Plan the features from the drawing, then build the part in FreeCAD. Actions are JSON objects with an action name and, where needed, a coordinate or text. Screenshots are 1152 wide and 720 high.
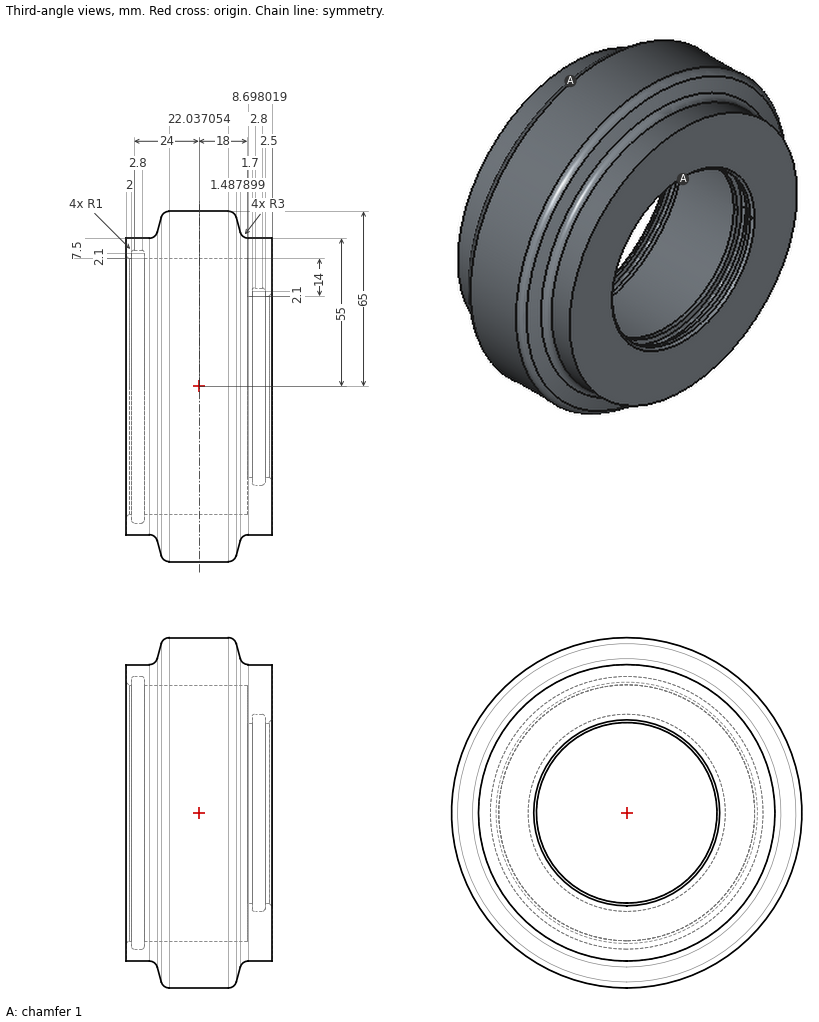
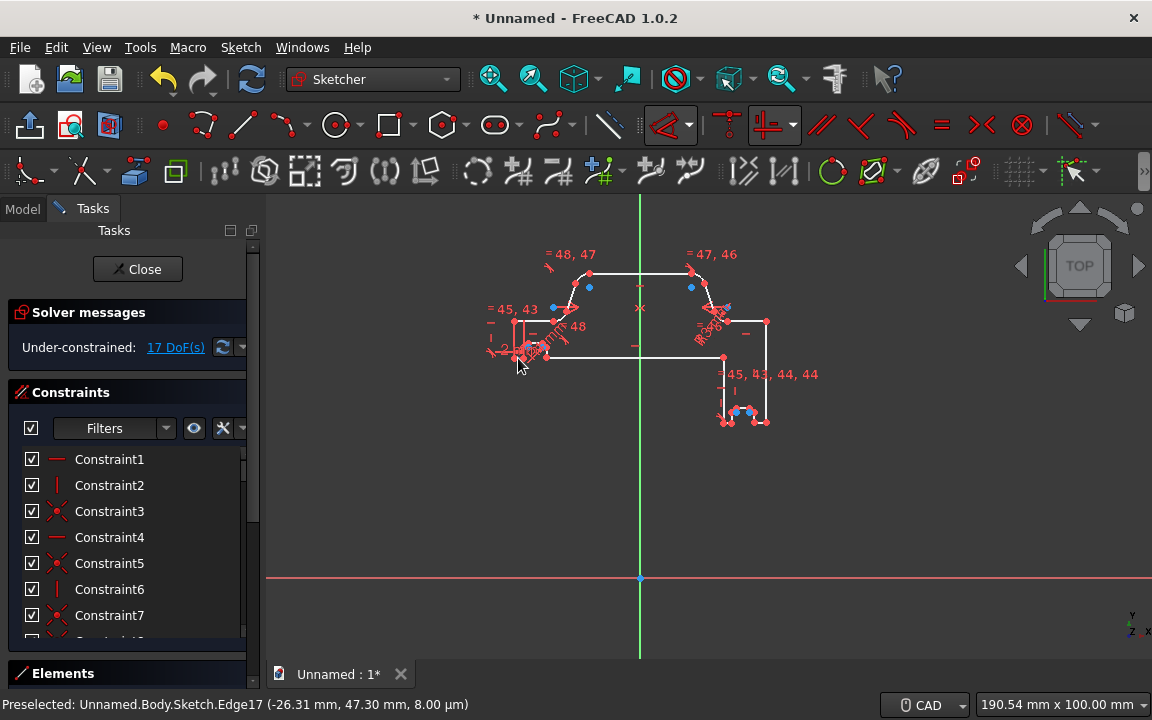
{"action": "scroll", "coordinate": [724, 377], "scroll_direction": "up", "scroll_amount": 4}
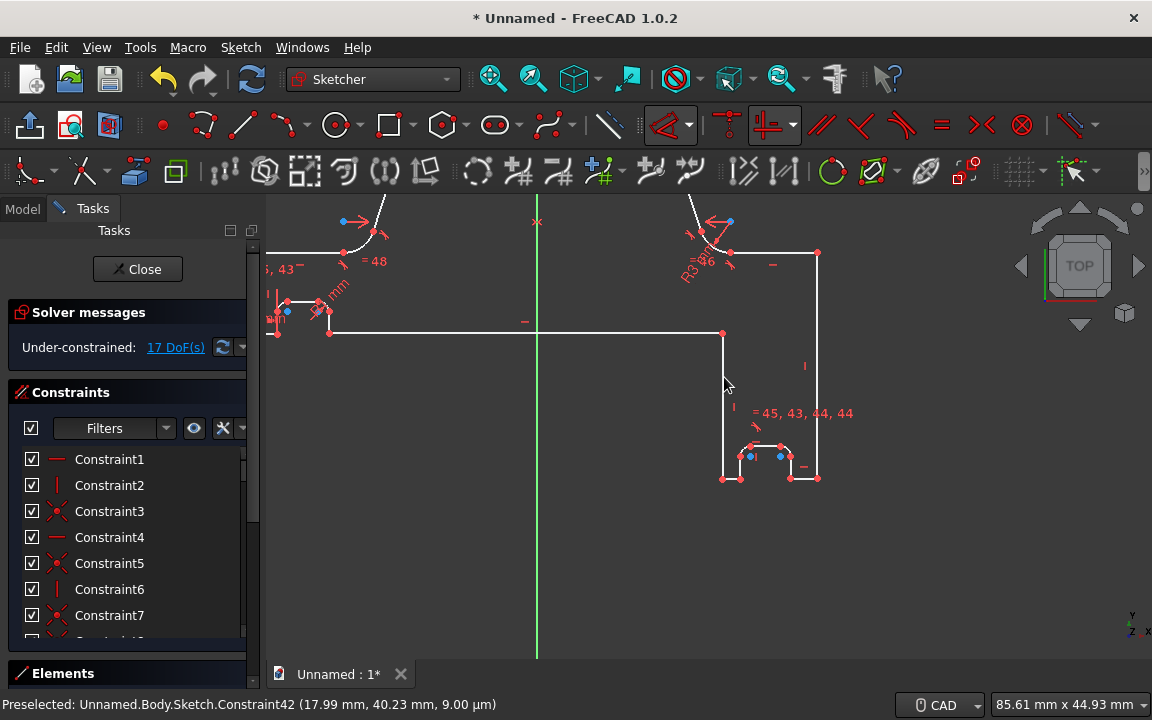
{"action": "left_click", "coordinate": [723, 377]}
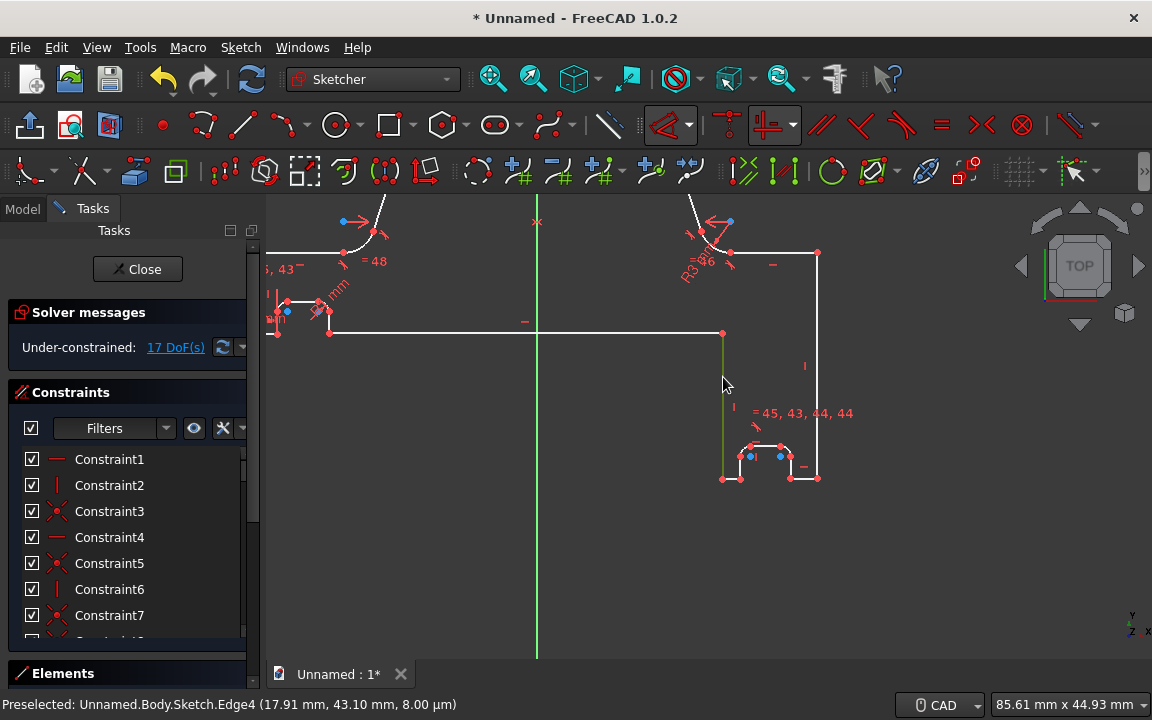
{"action": "key", "text": "i"}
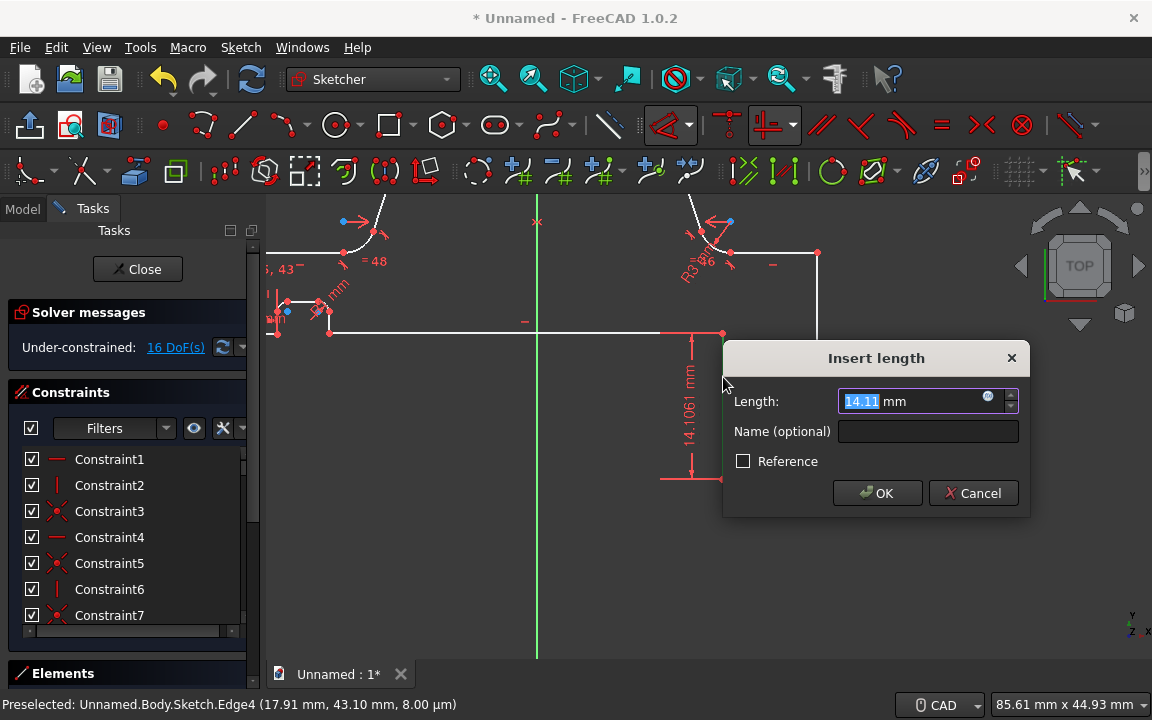
{"action": "type", "text": "14"}
{"action": "key", "text": "Return"}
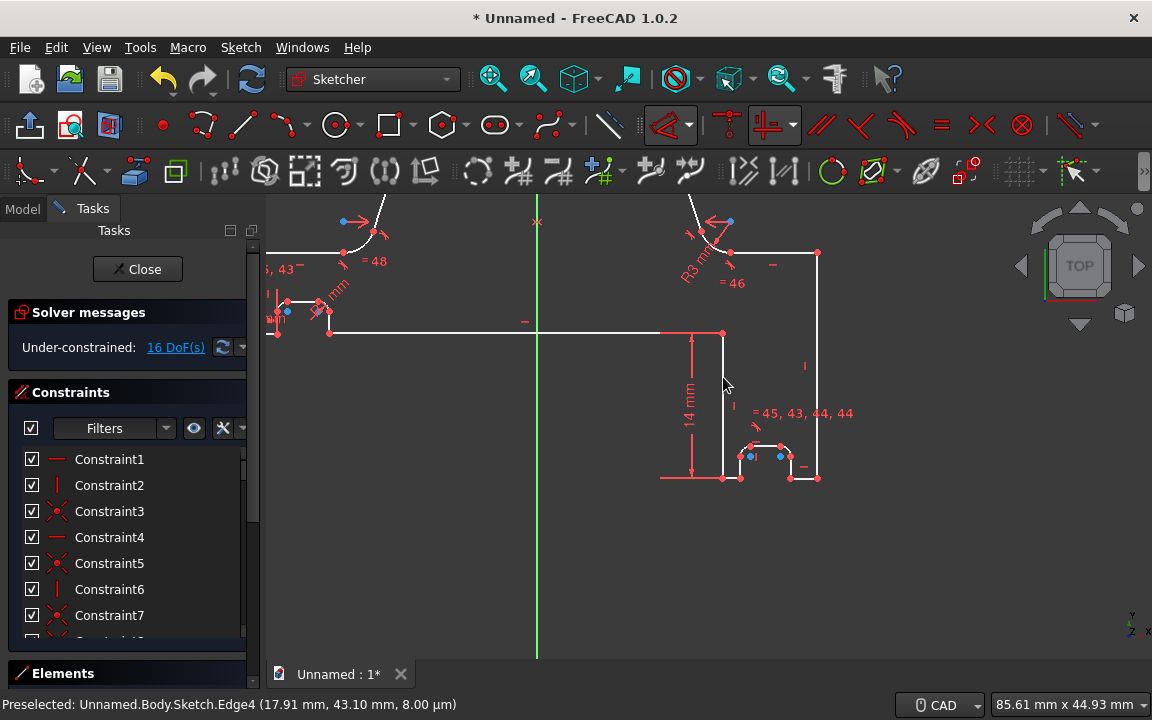
{"action": "scroll", "coordinate": [297, 302], "scroll_direction": "up", "scroll_amount": 2}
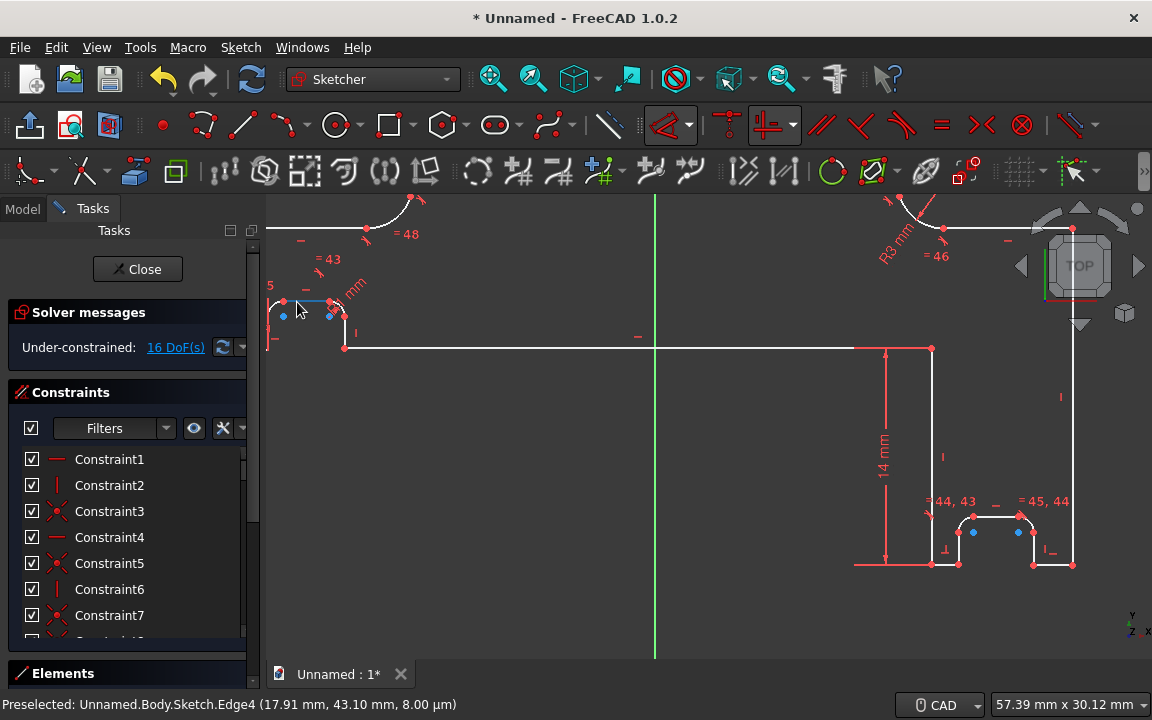
{"action": "left_click", "coordinate": [297, 301]}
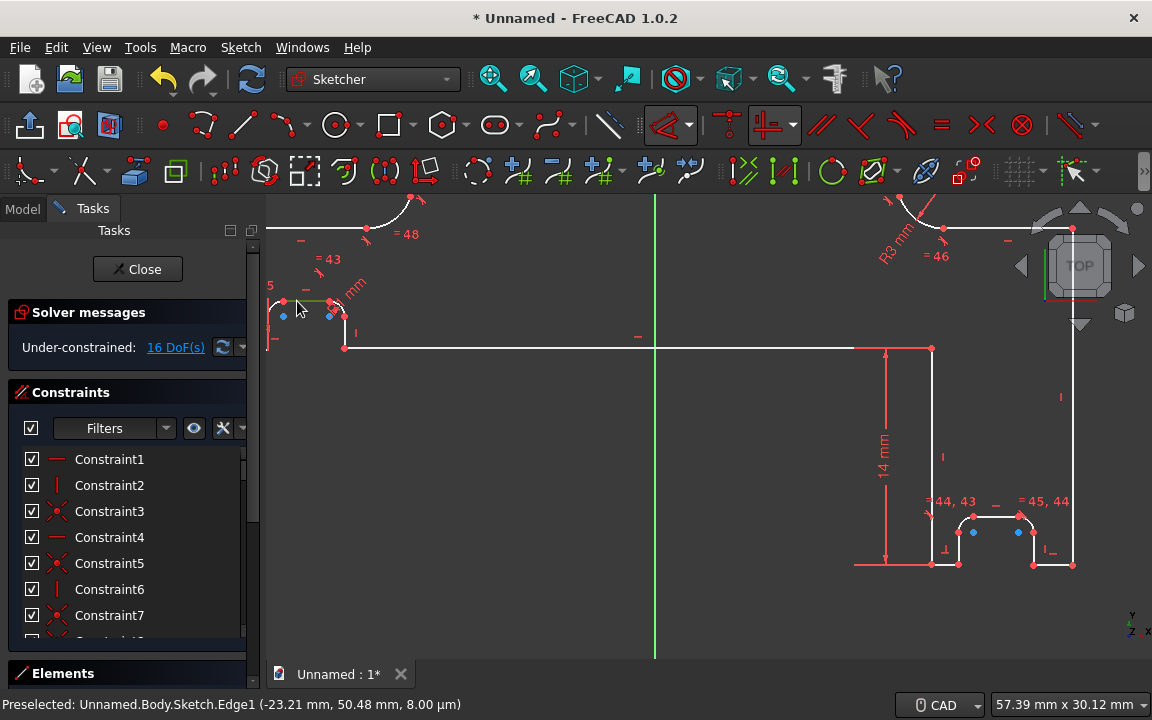
{"action": "key", "text": "l"}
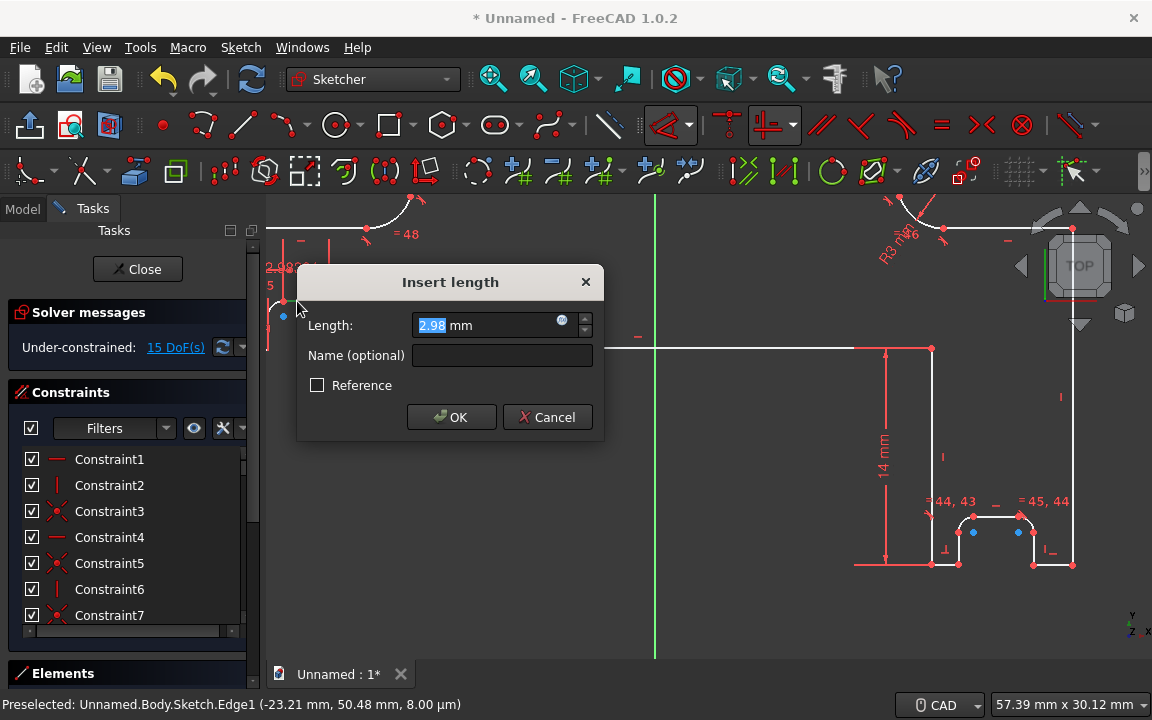
{"action": "type", "text": "2.8"}
{"action": "key", "text": "Return"}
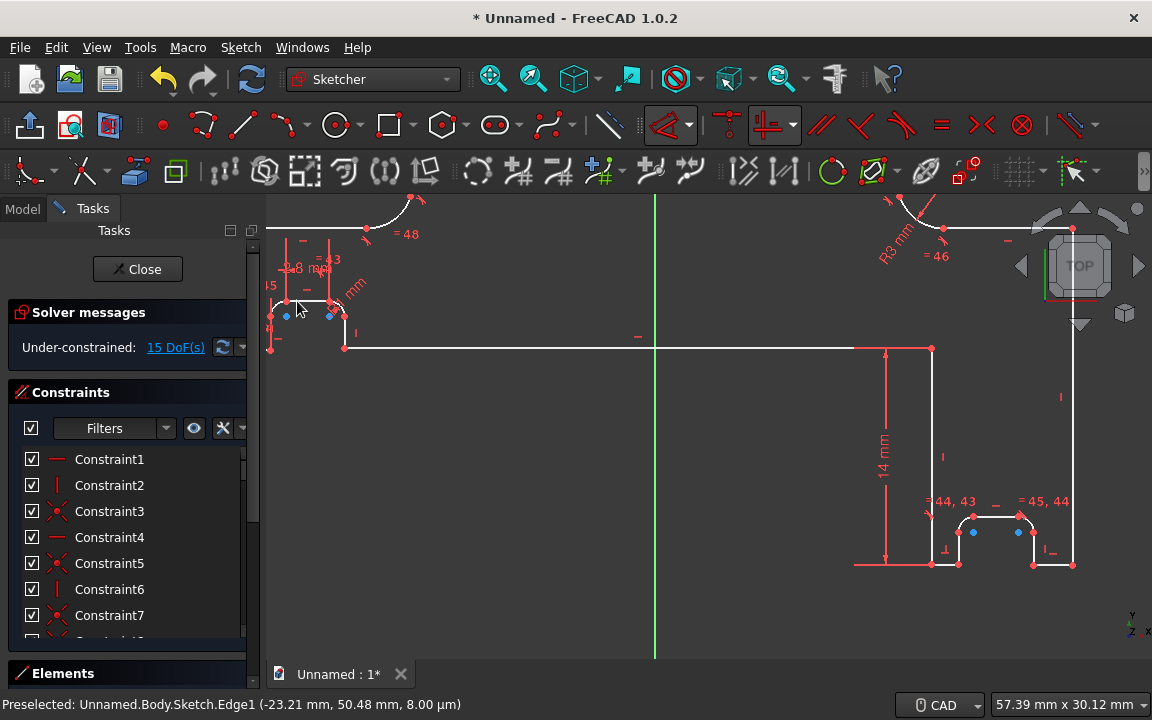
{"action": "scroll", "coordinate": [345, 326], "scroll_direction": "up", "scroll_amount": 2}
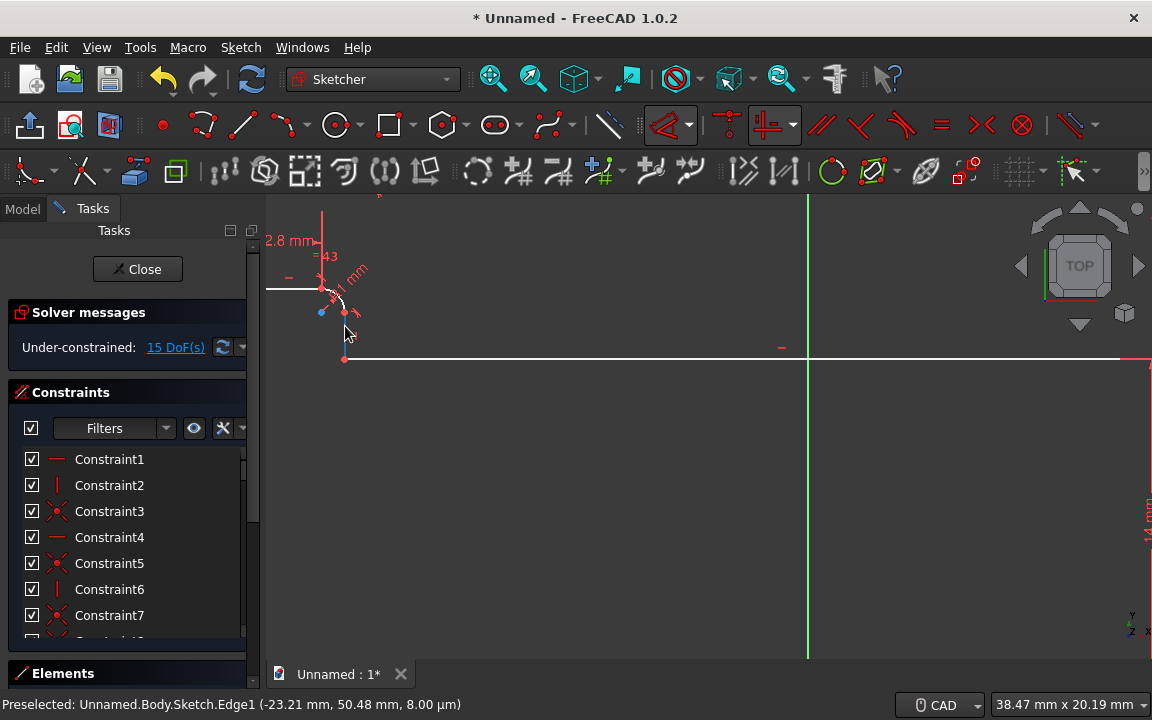
{"action": "left_click", "coordinate": [345, 326]}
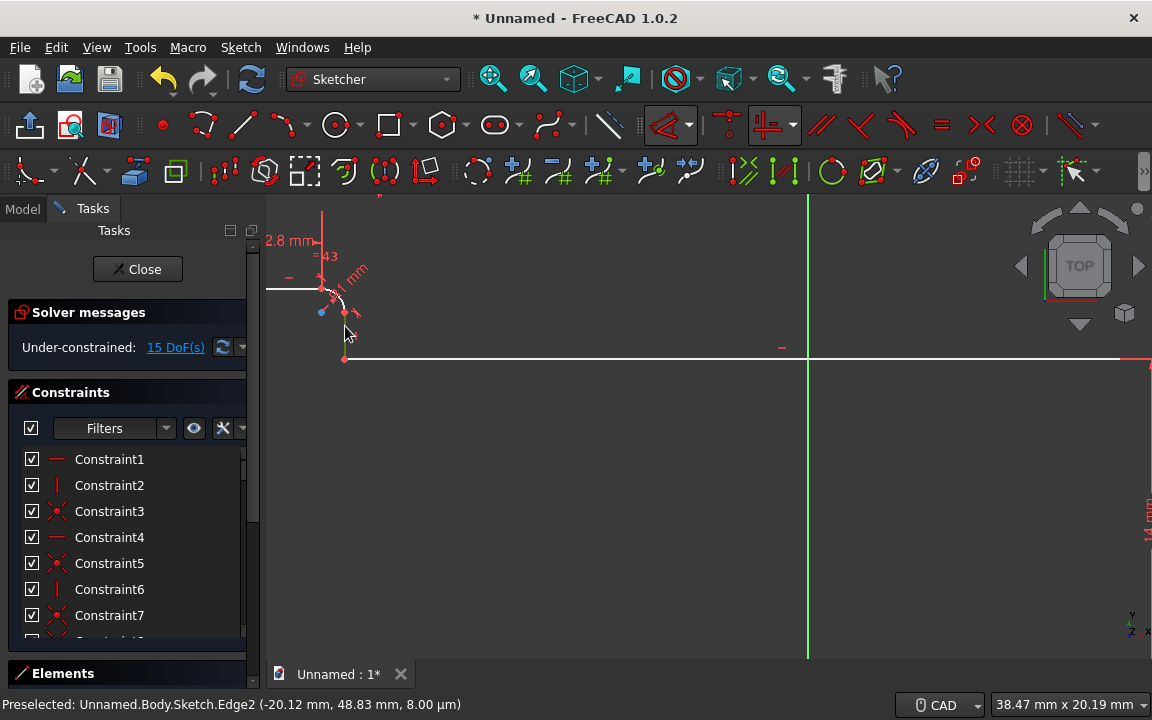
{"action": "left_click", "coordinate": [692, 126]}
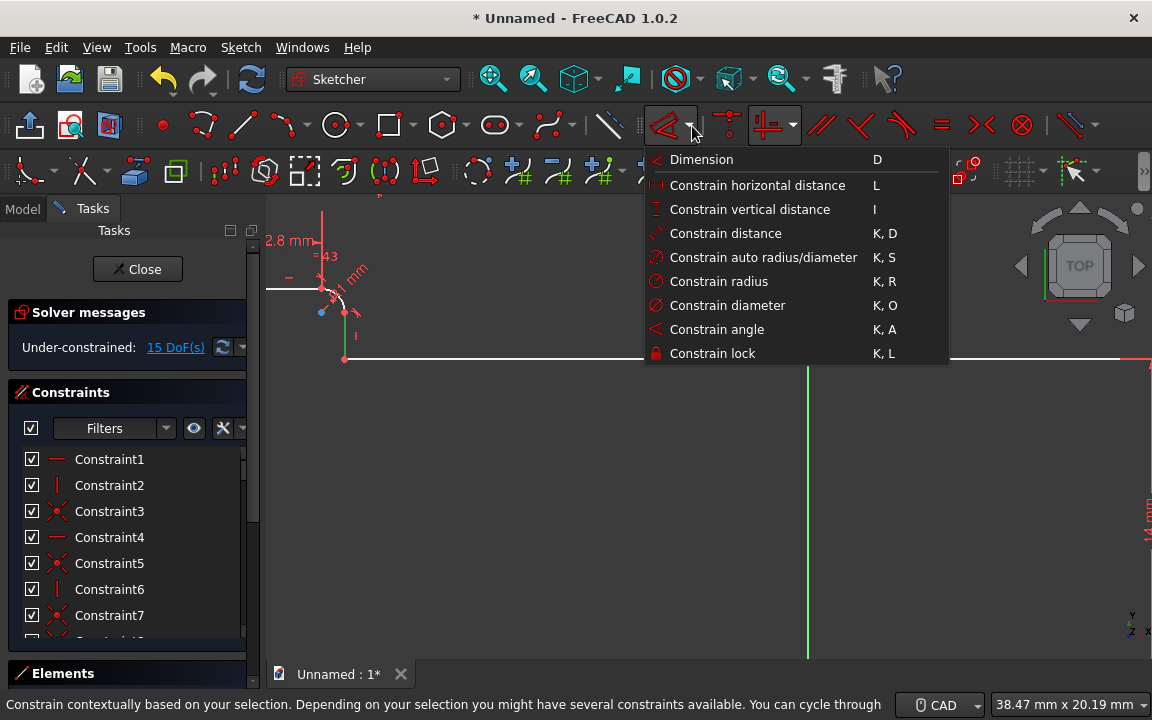
{"action": "left_click", "coordinate": [797, 209]}